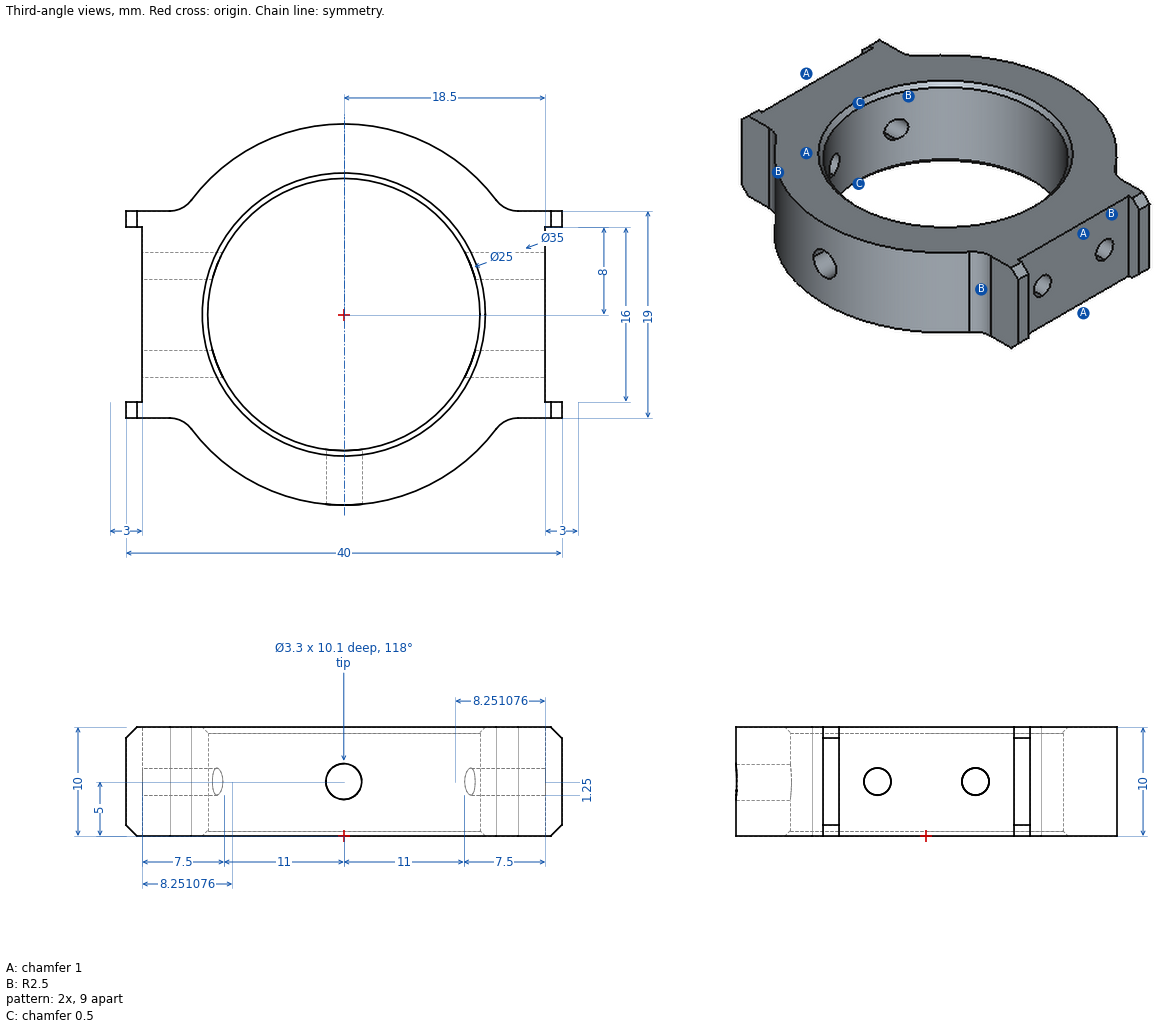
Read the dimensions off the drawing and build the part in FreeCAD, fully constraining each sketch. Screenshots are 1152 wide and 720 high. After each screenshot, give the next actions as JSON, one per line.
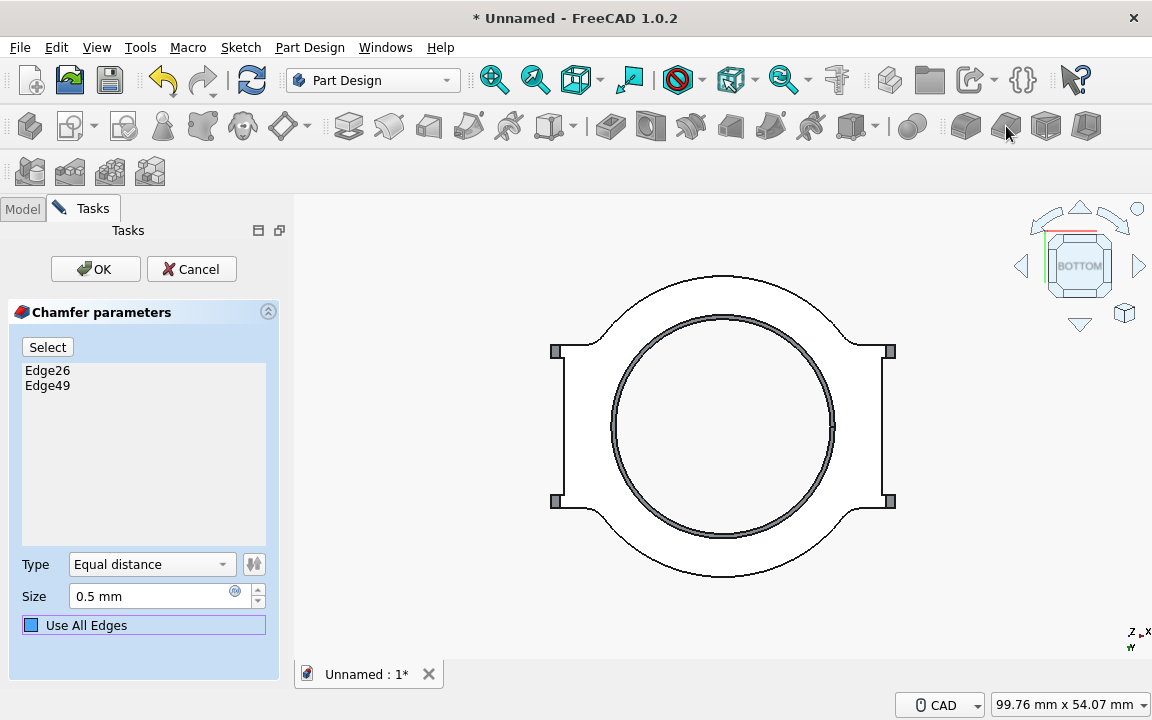
{"action": "left_click", "coordinate": [96, 269]}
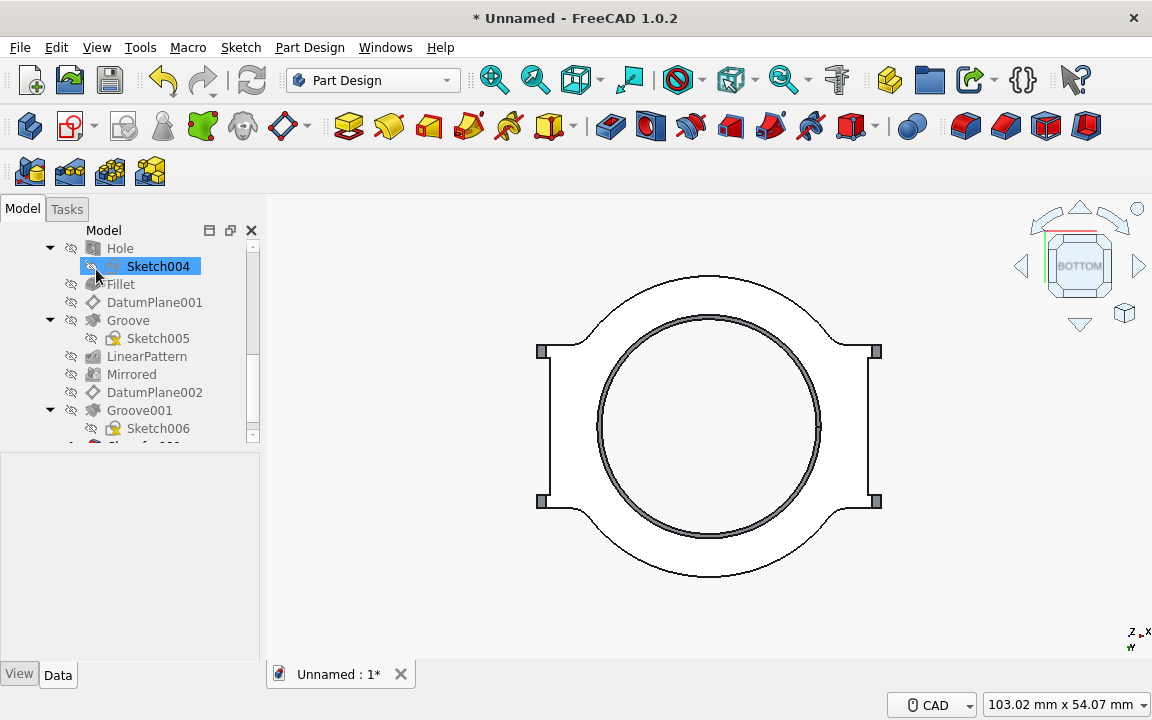
{"action": "key", "text": "0"}